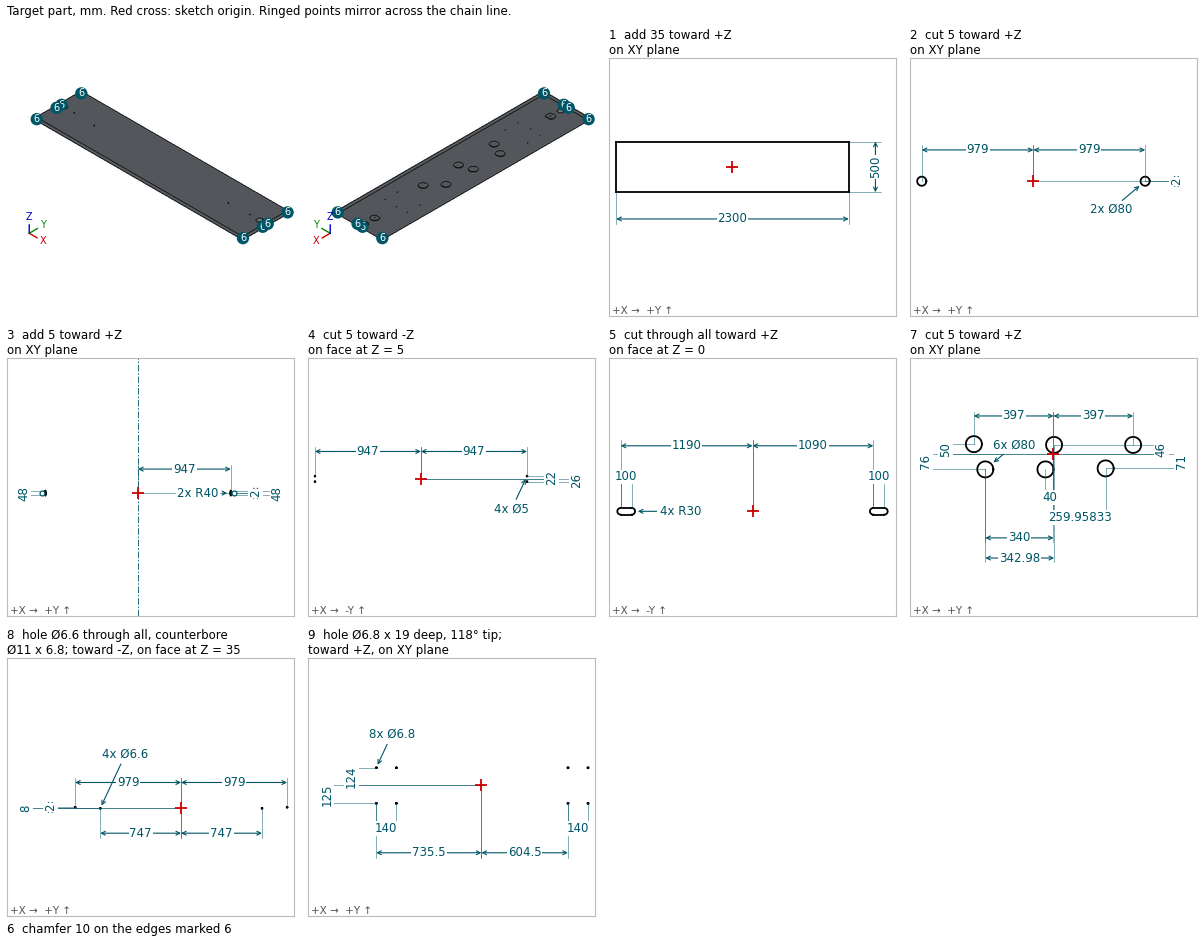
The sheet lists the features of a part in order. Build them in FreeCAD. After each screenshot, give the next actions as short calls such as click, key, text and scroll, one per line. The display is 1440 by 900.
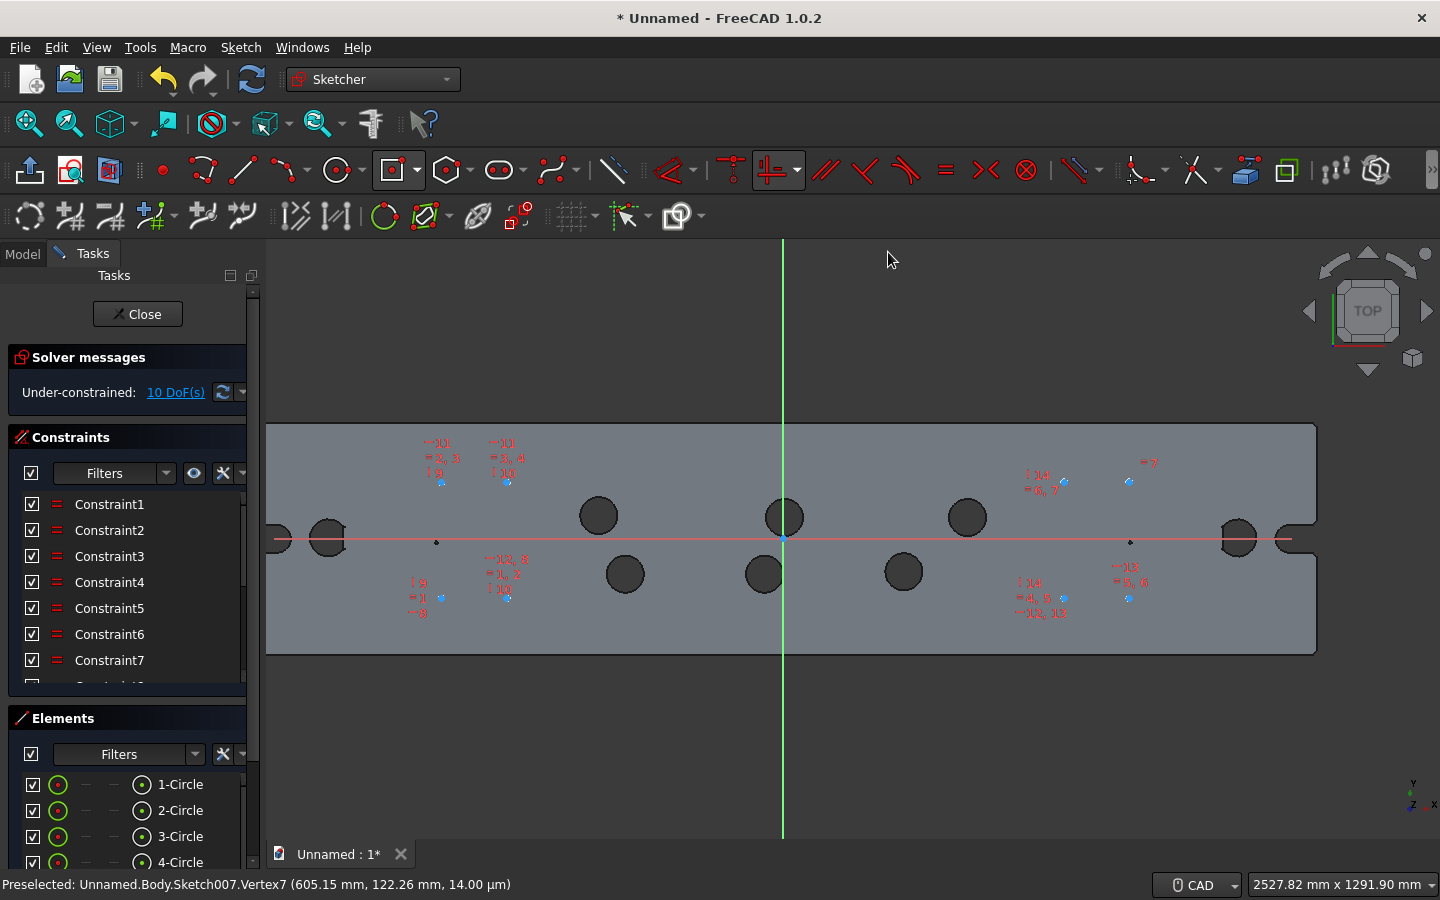
click(507, 483)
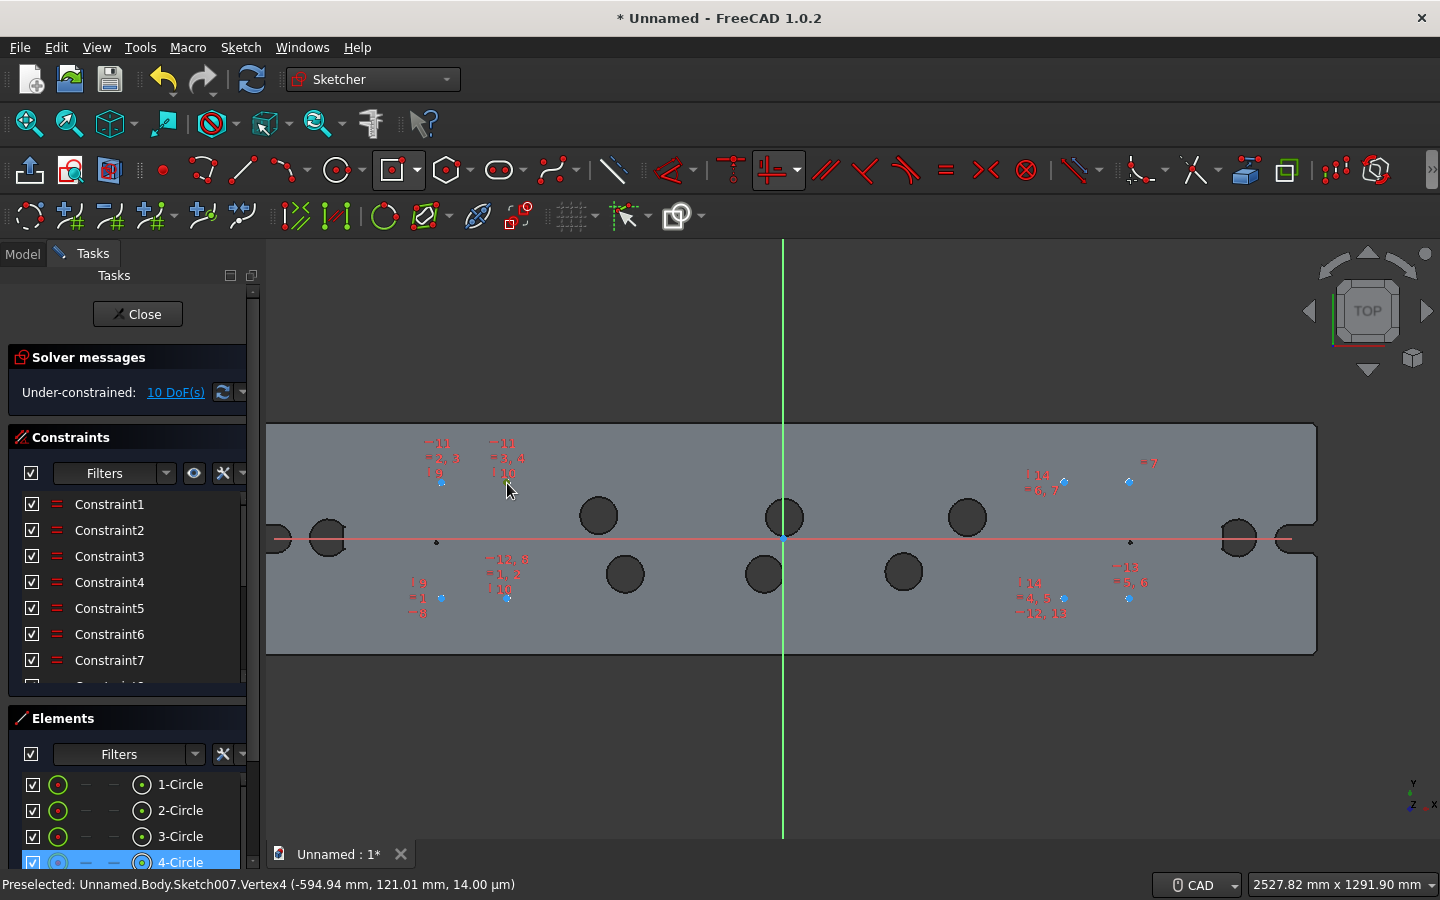
click(1064, 482)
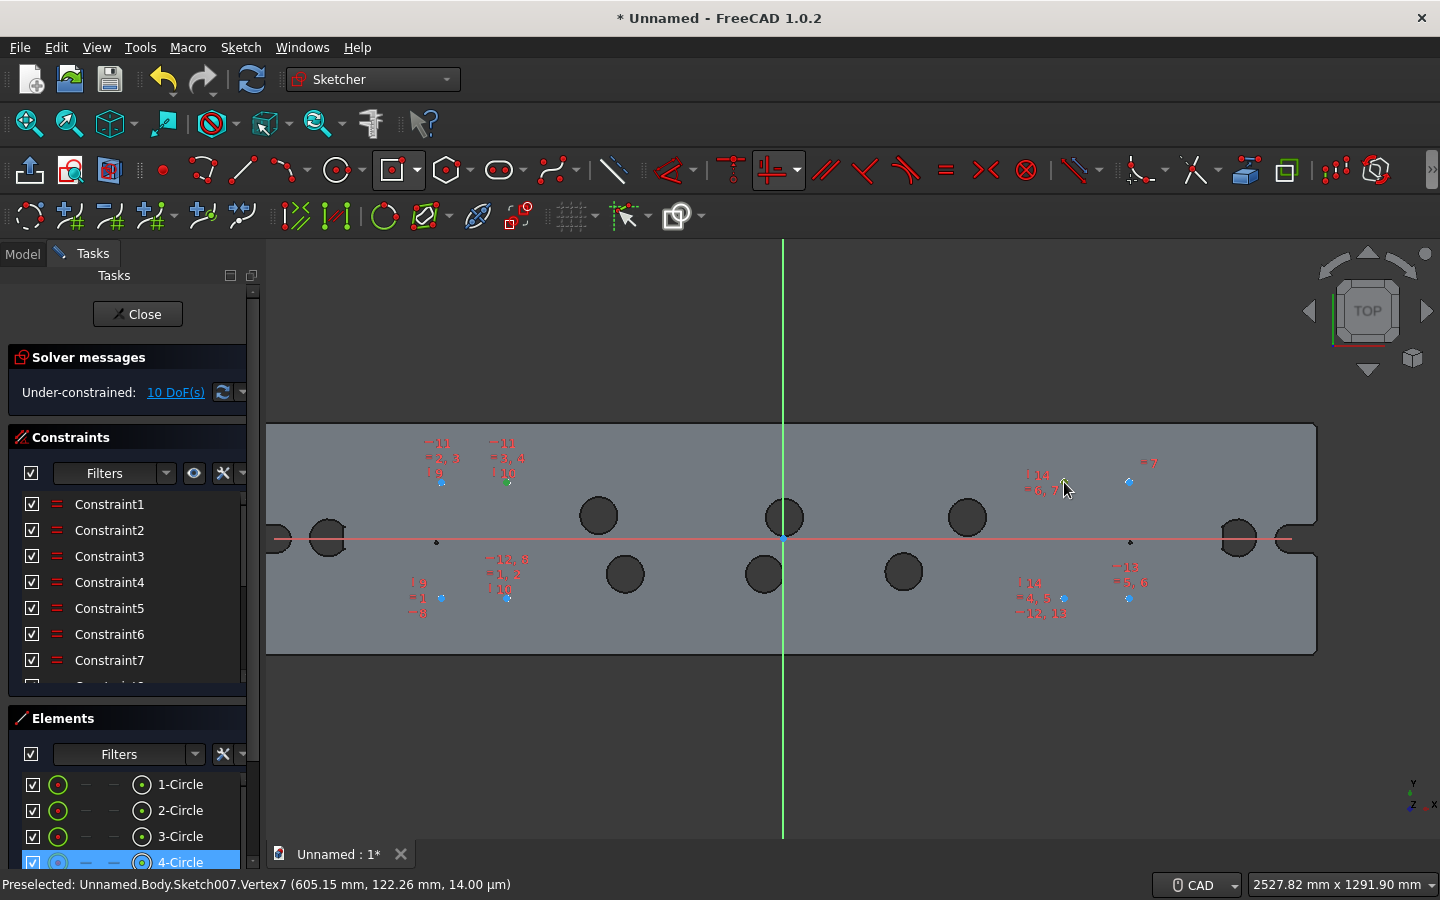
key(h)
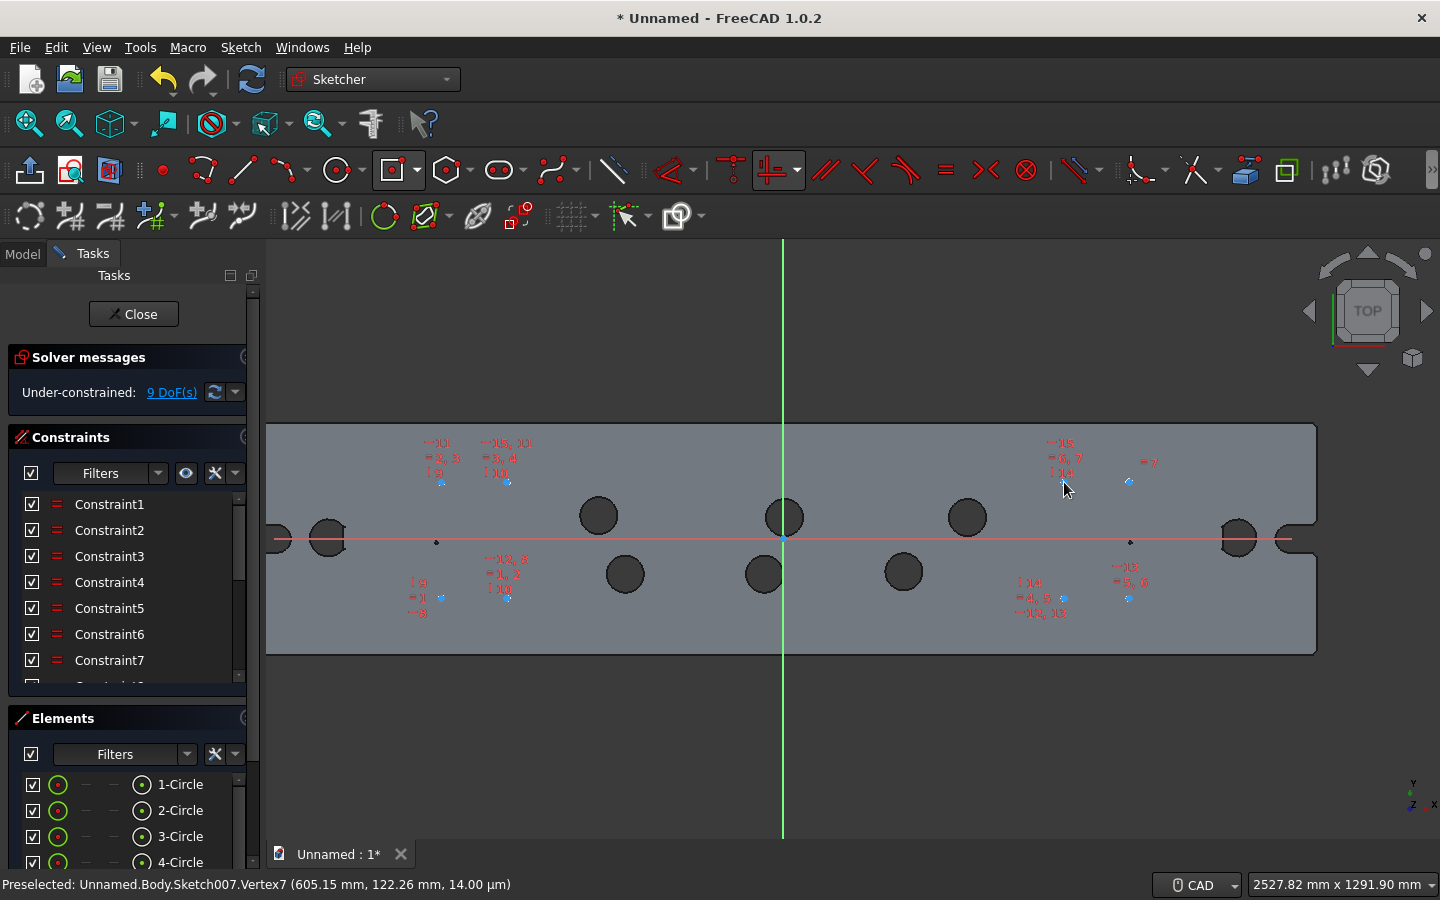
click(1129, 598)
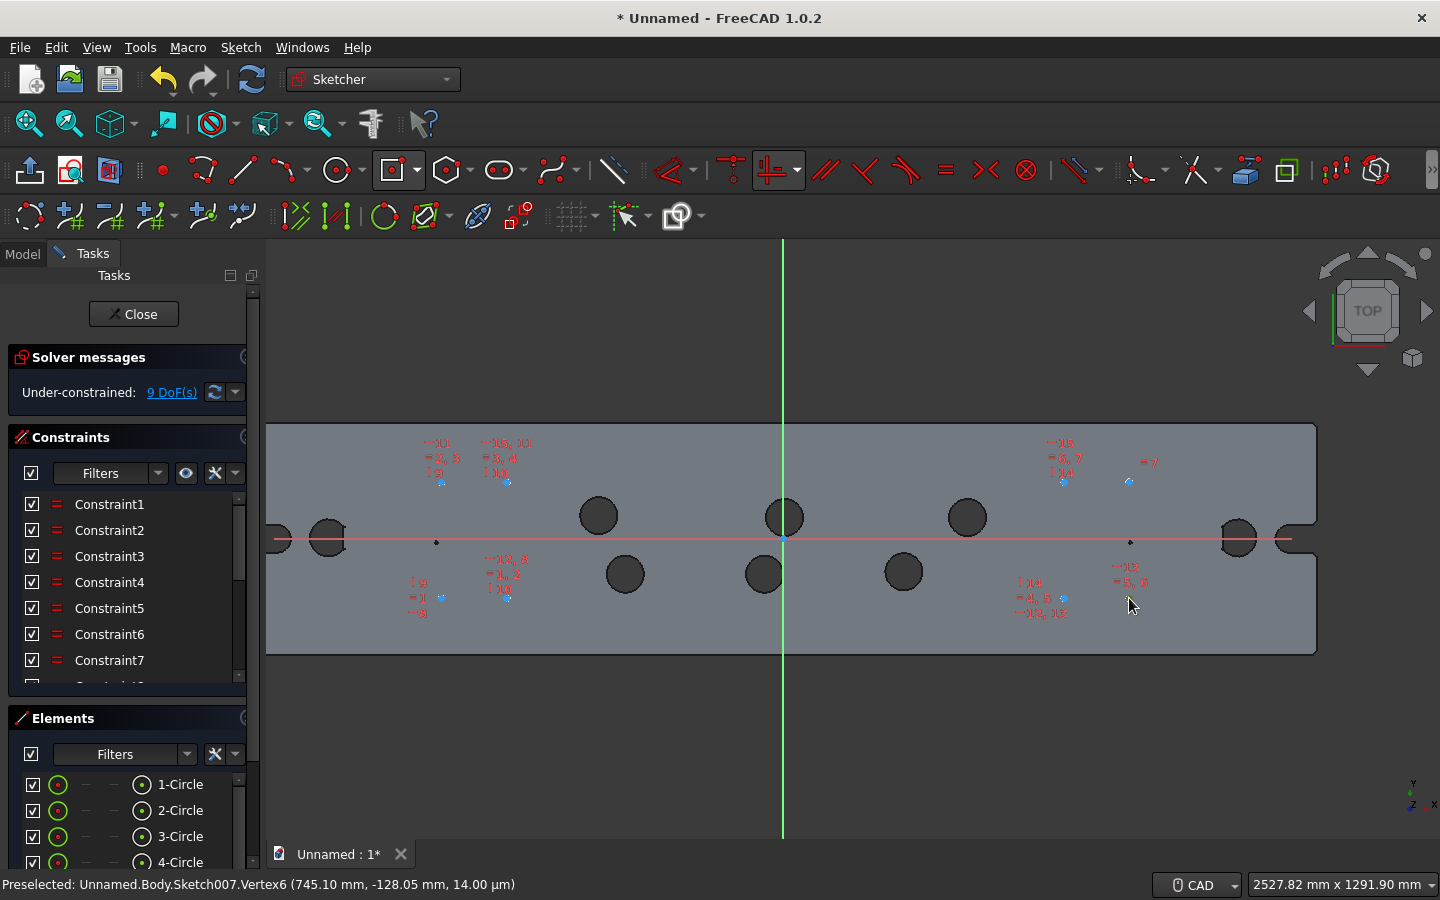
click(1129, 482)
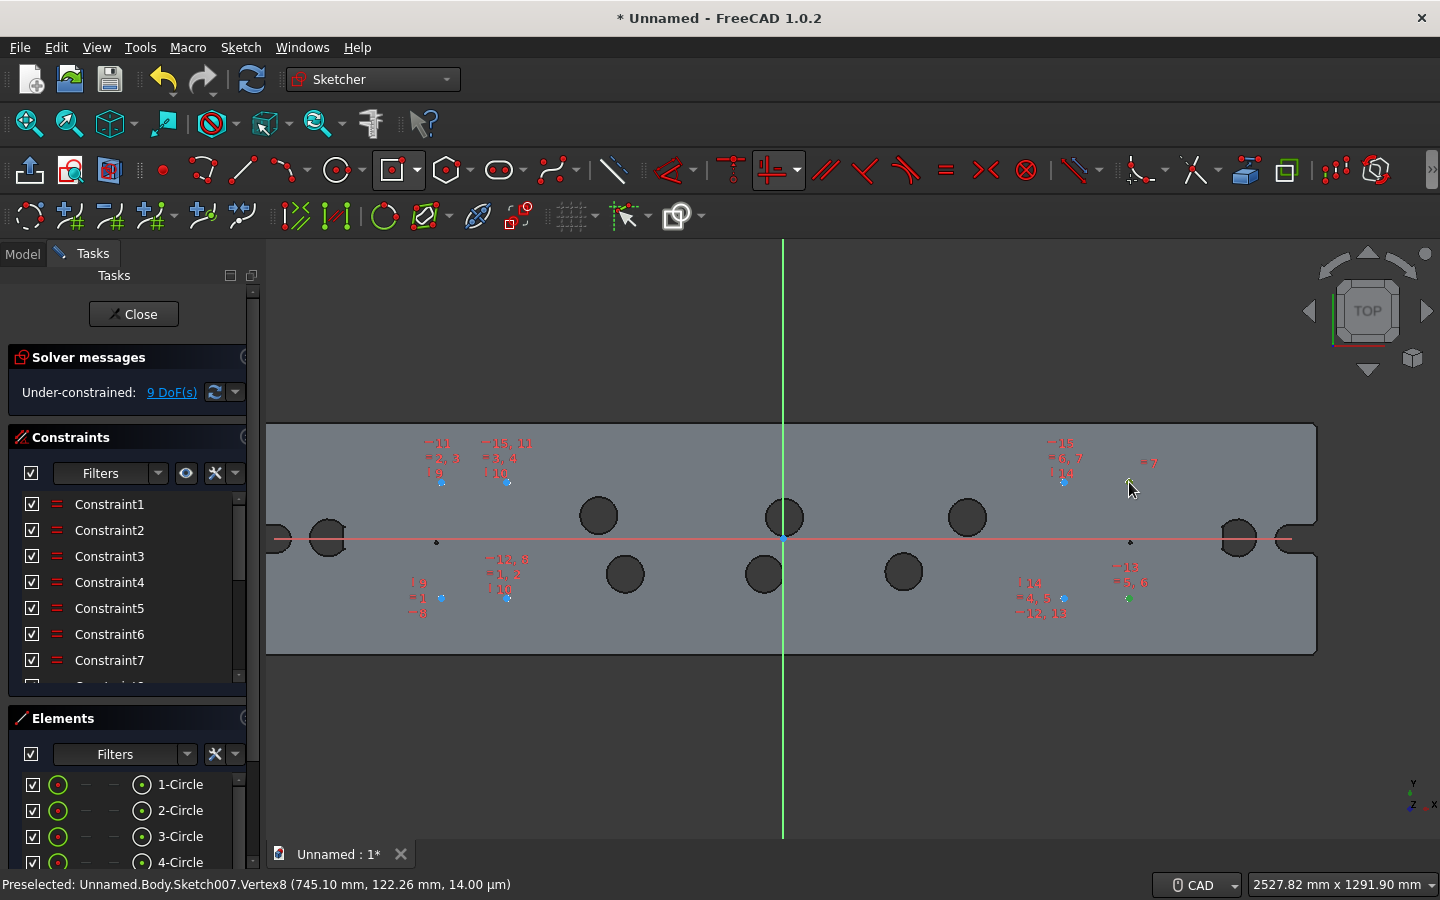
key(v)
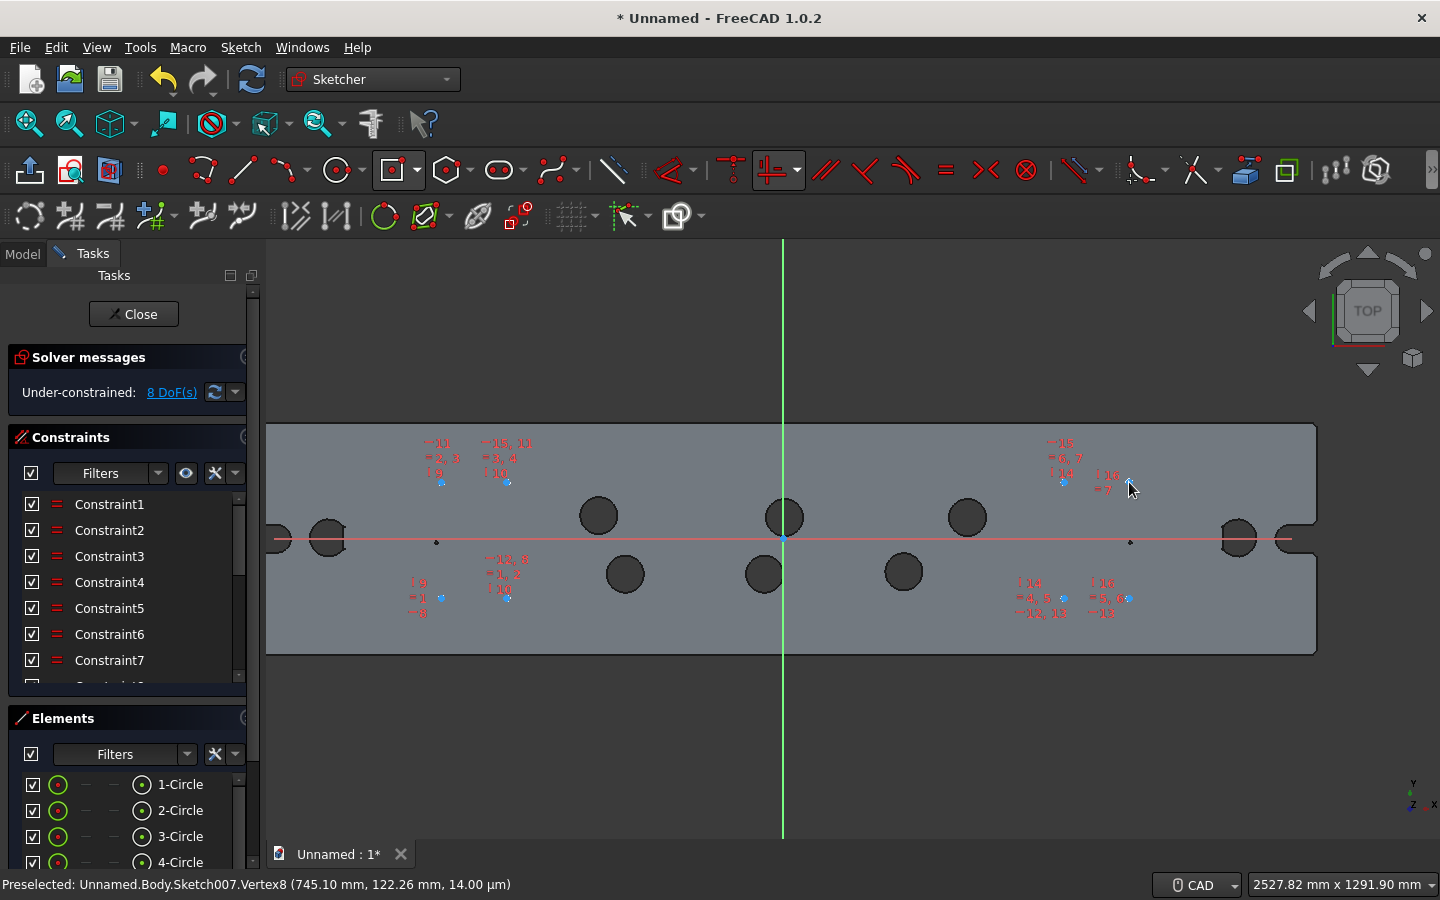
click(1064, 483)